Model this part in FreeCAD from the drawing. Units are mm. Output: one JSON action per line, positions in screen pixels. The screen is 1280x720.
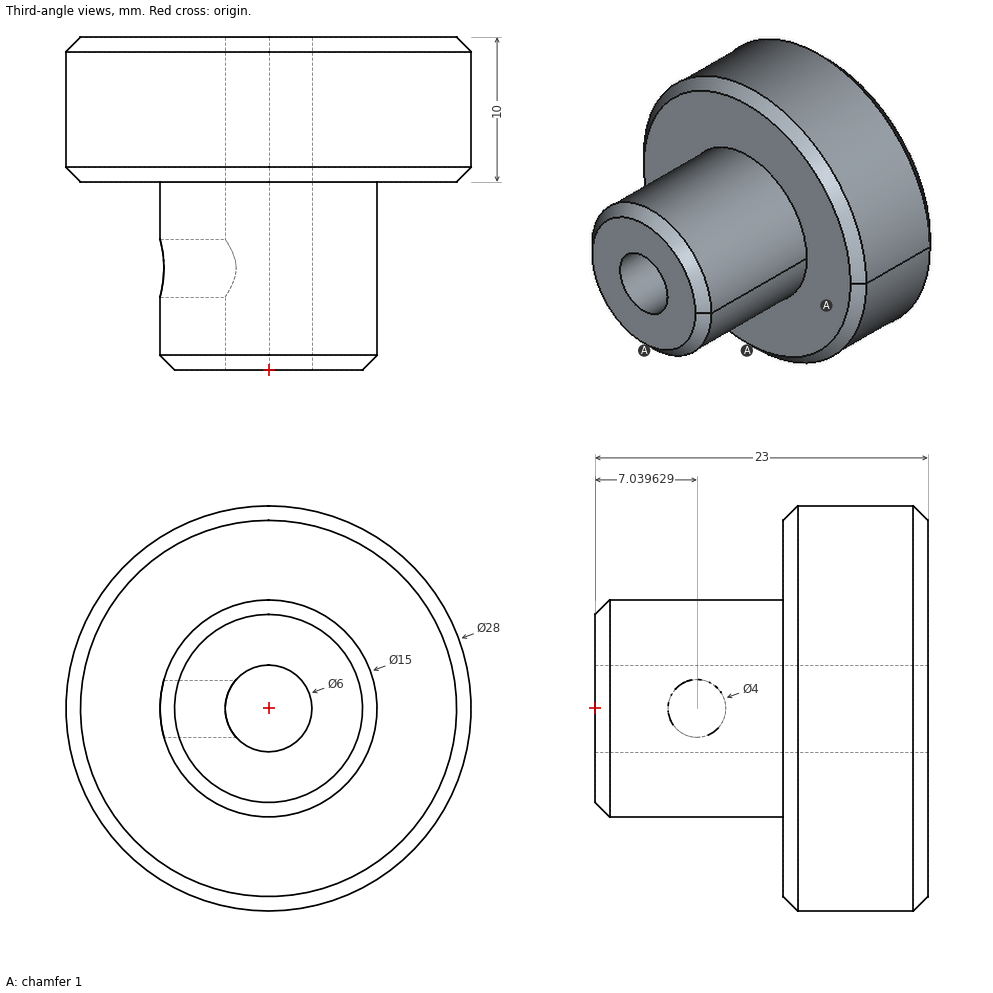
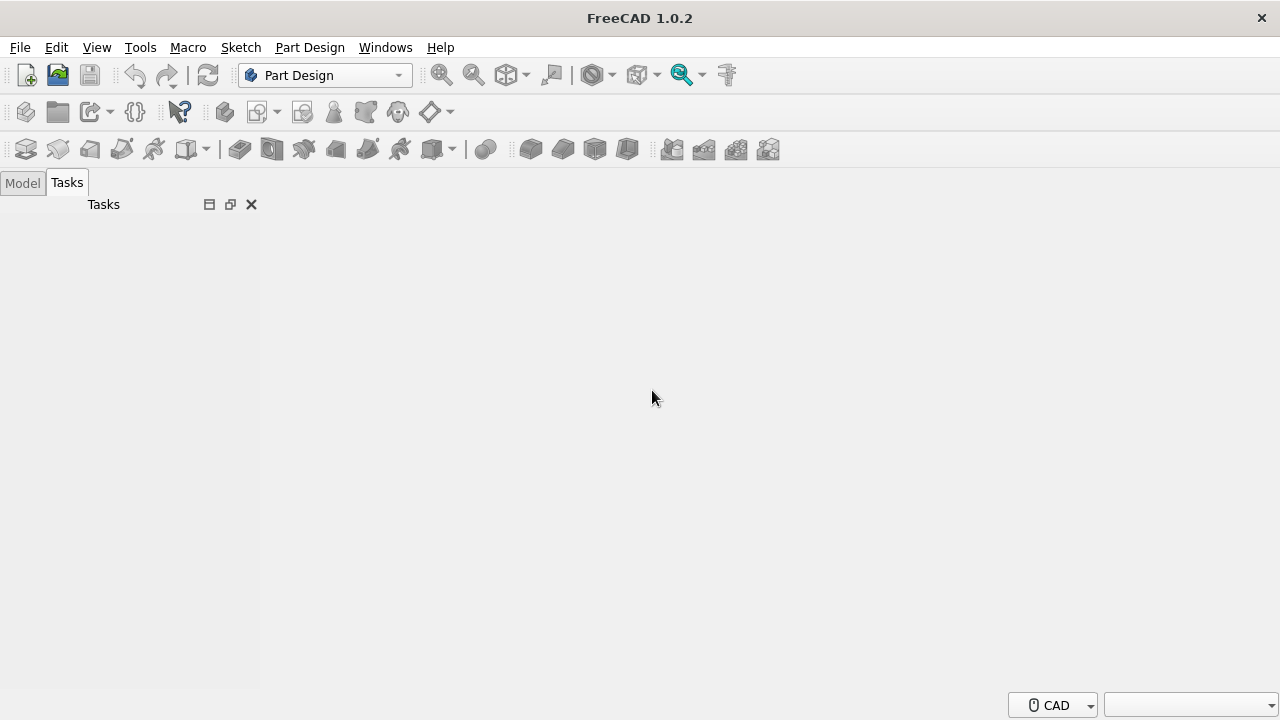
{"action": "left_click", "coordinate": [26, 76]}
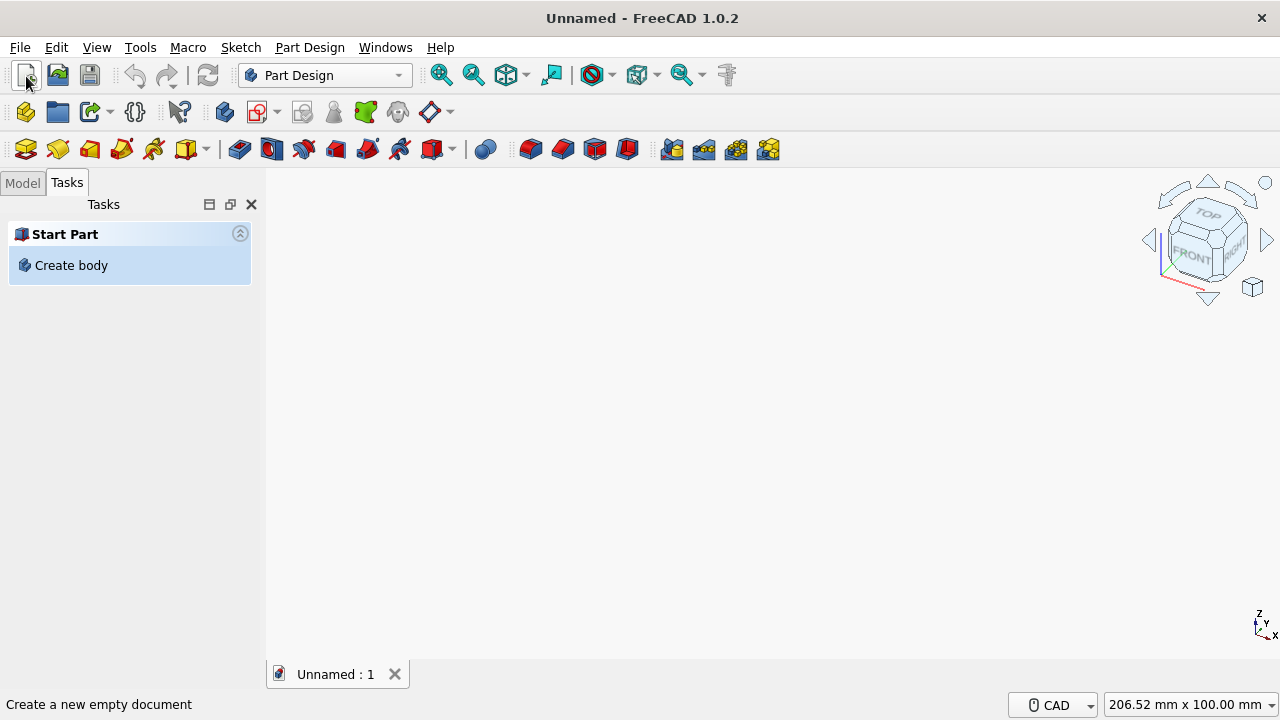
{"action": "left_click", "coordinate": [258, 112]}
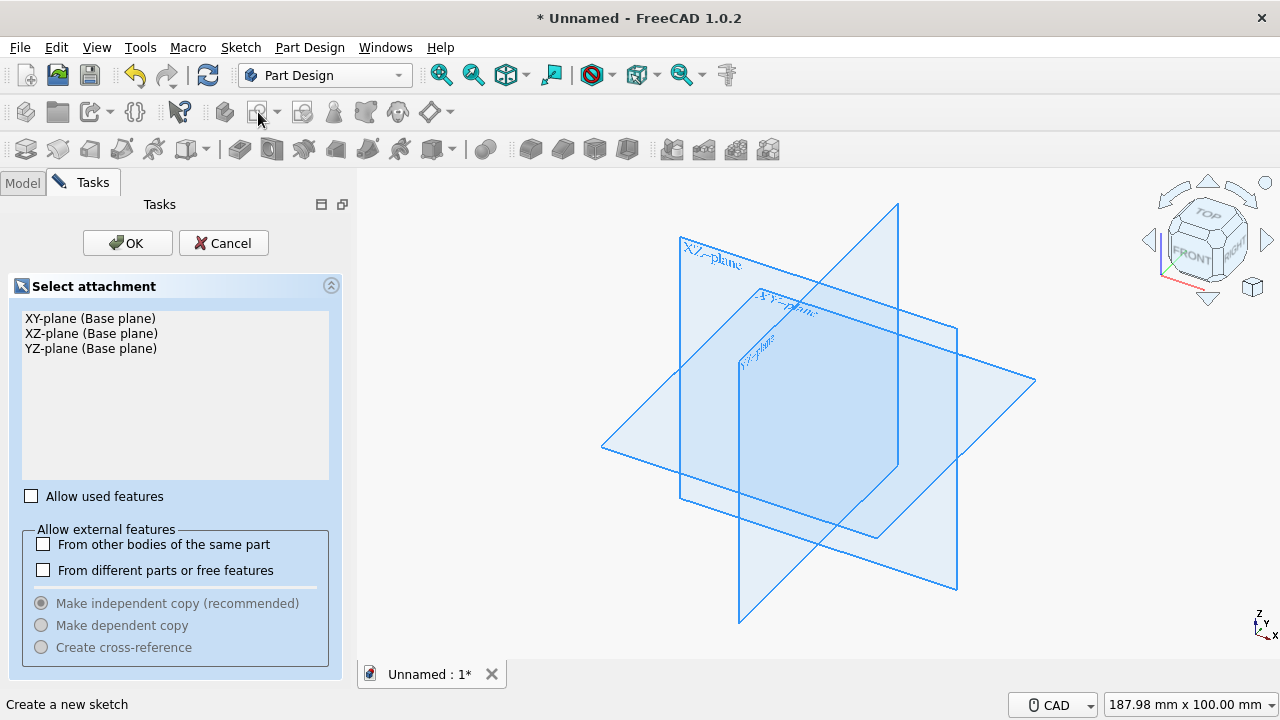
{"action": "left_click", "coordinate": [82, 334]}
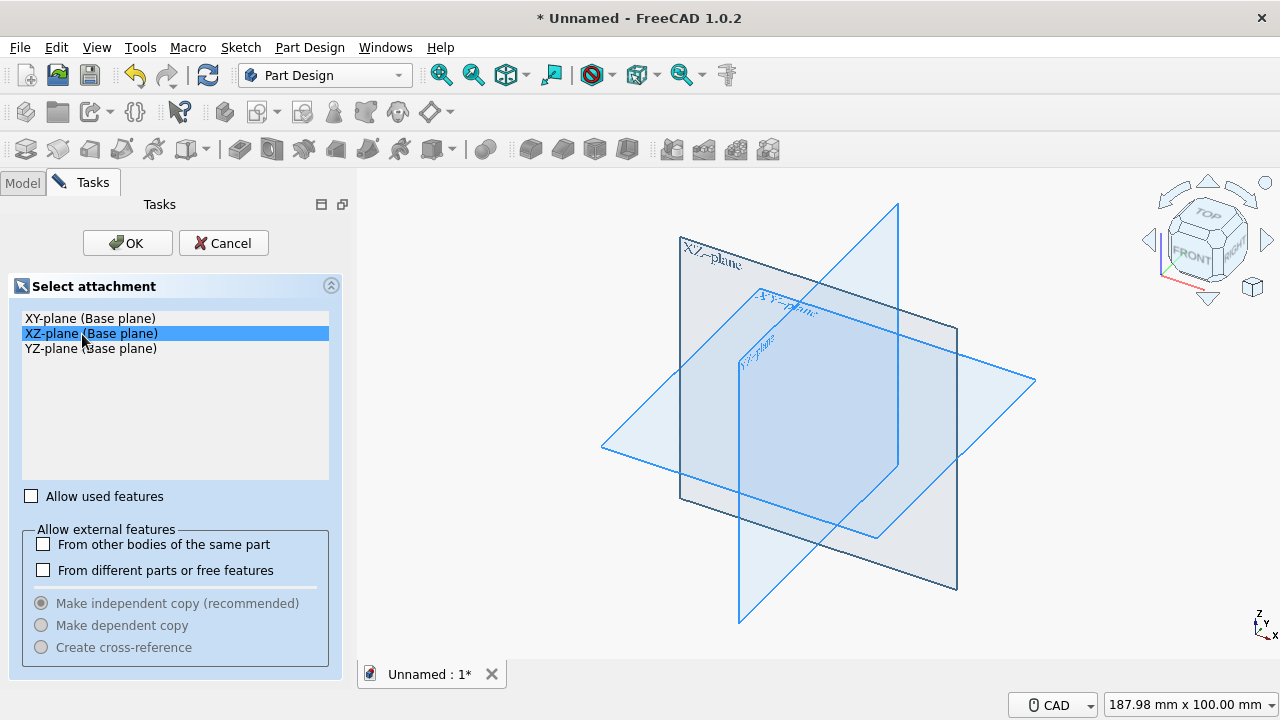
{"action": "left_click", "coordinate": [128, 243]}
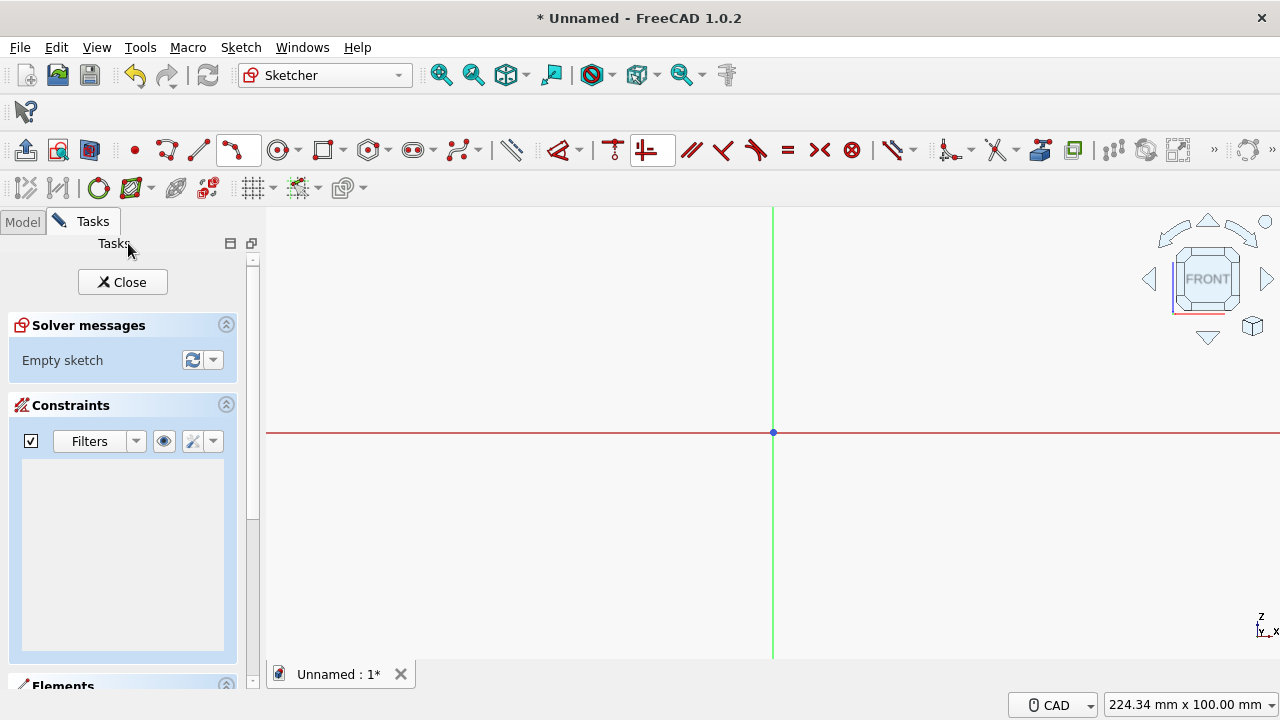
{"action": "scroll", "coordinate": [795, 433], "scroll_direction": "up", "scroll_amount": 7}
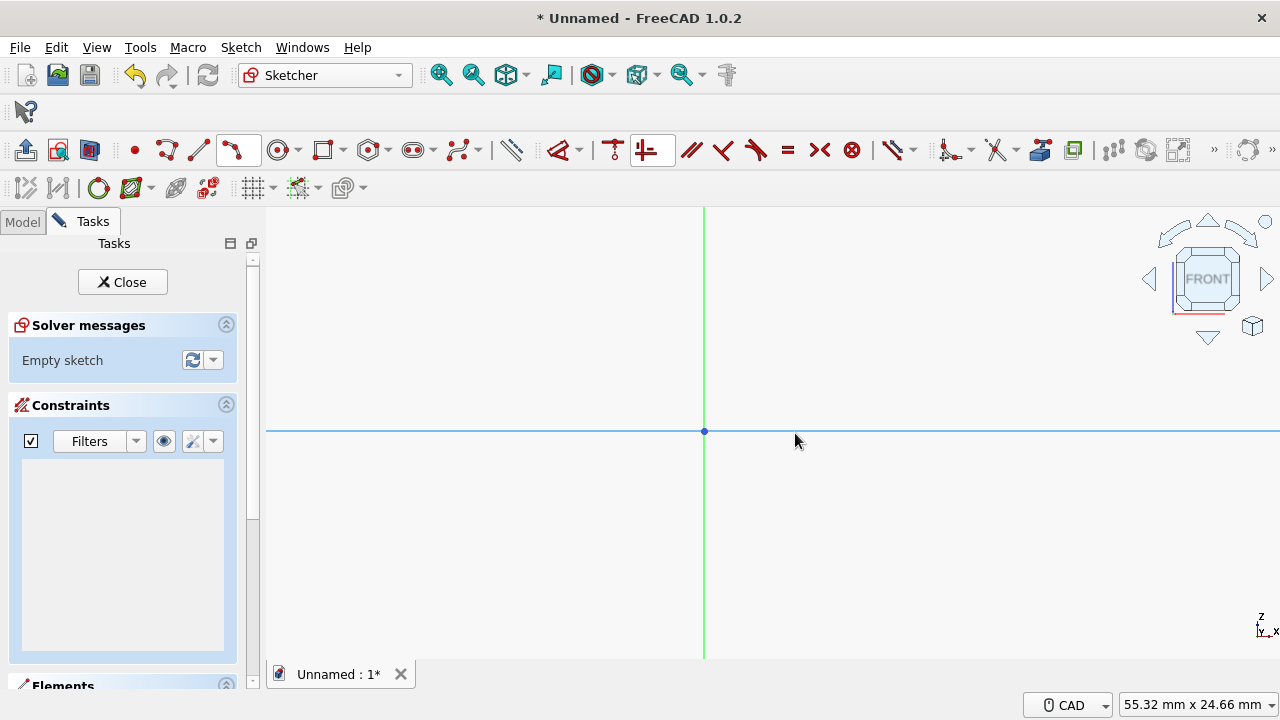
{"action": "left_click", "coordinate": [278, 150]}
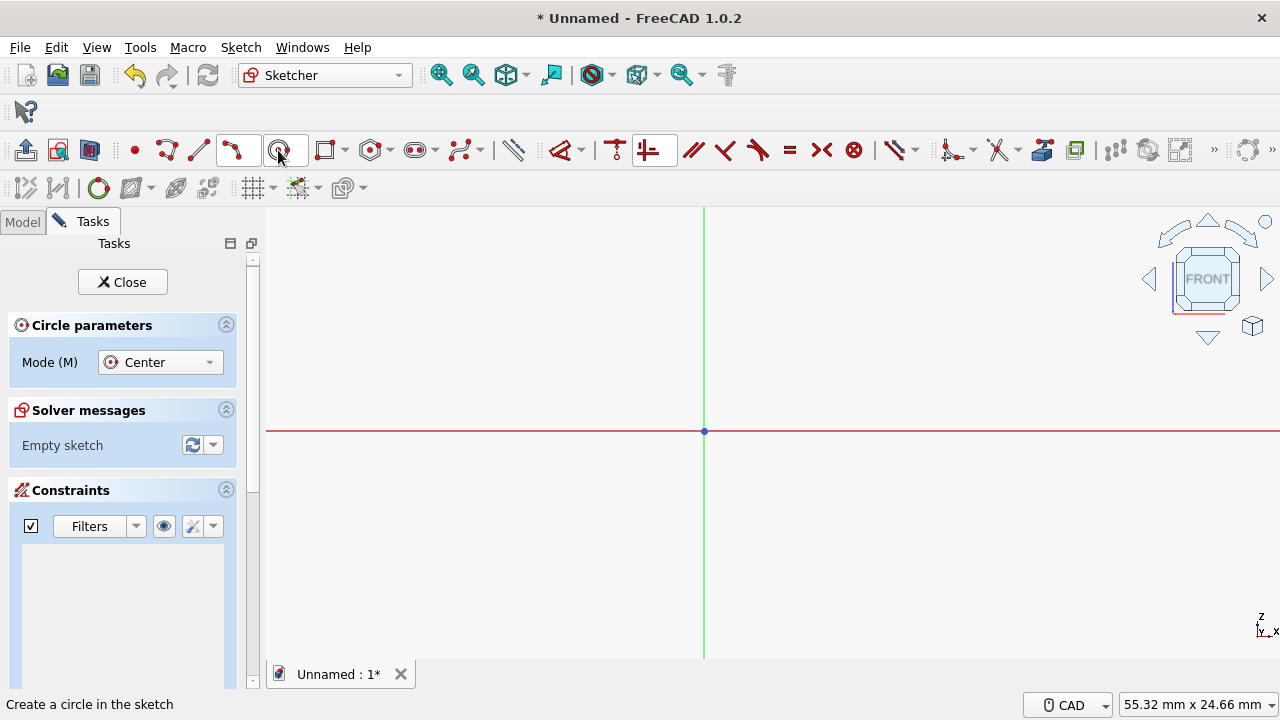
{"action": "left_click", "coordinate": [704, 431]}
{"action": "mouse_move", "coordinate": [801, 334]}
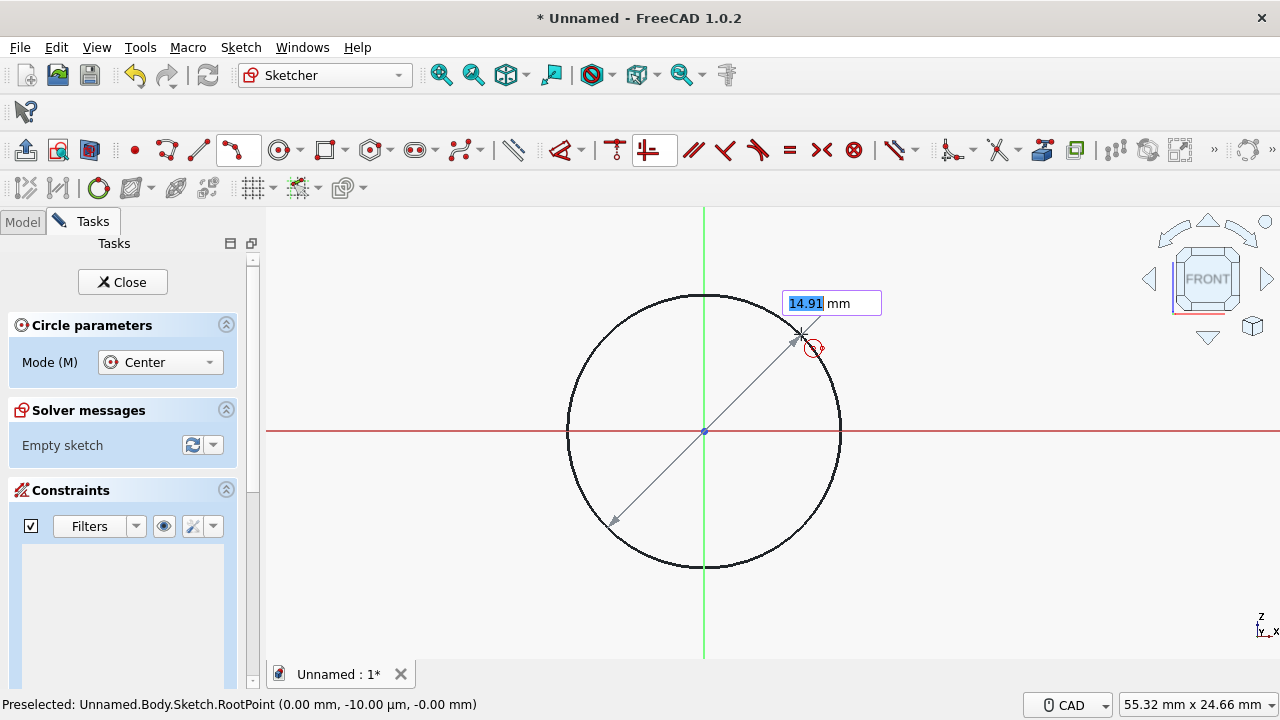
{"action": "type", "text": "15"}
{"action": "key", "text": "Return"}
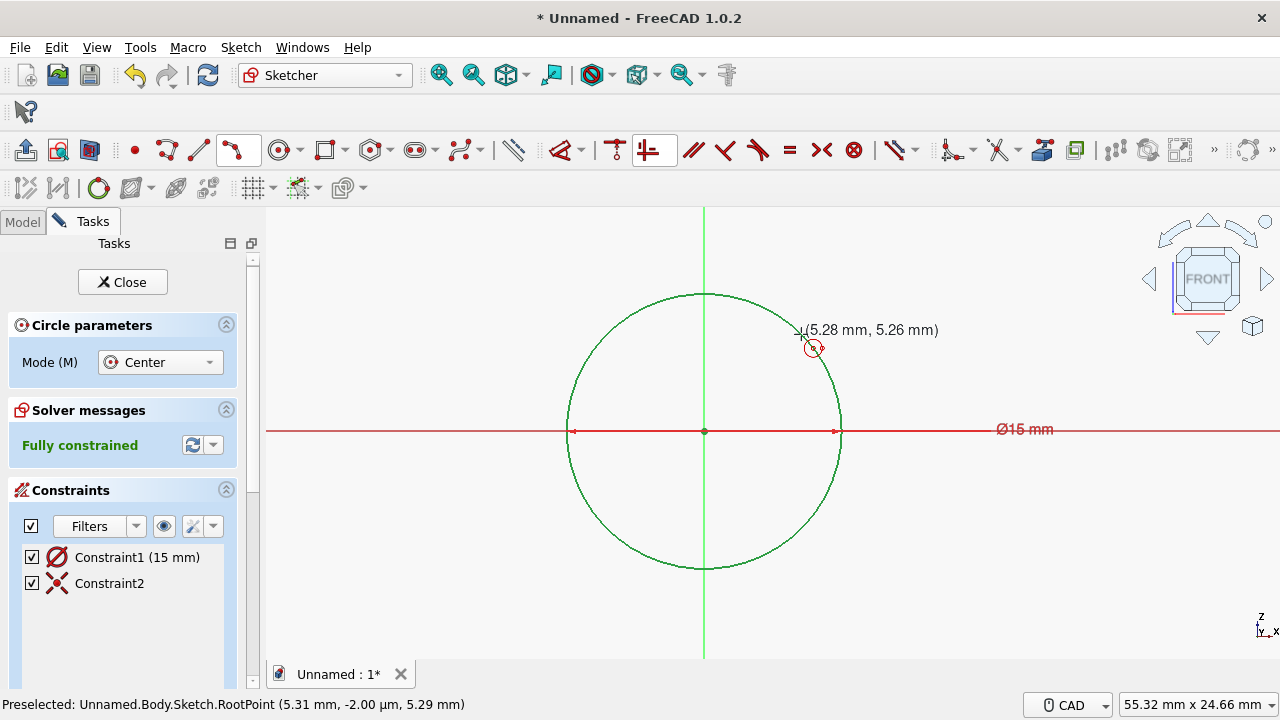
{"action": "left_click", "coordinate": [704, 431]}
{"action": "mouse_move", "coordinate": [743, 393]}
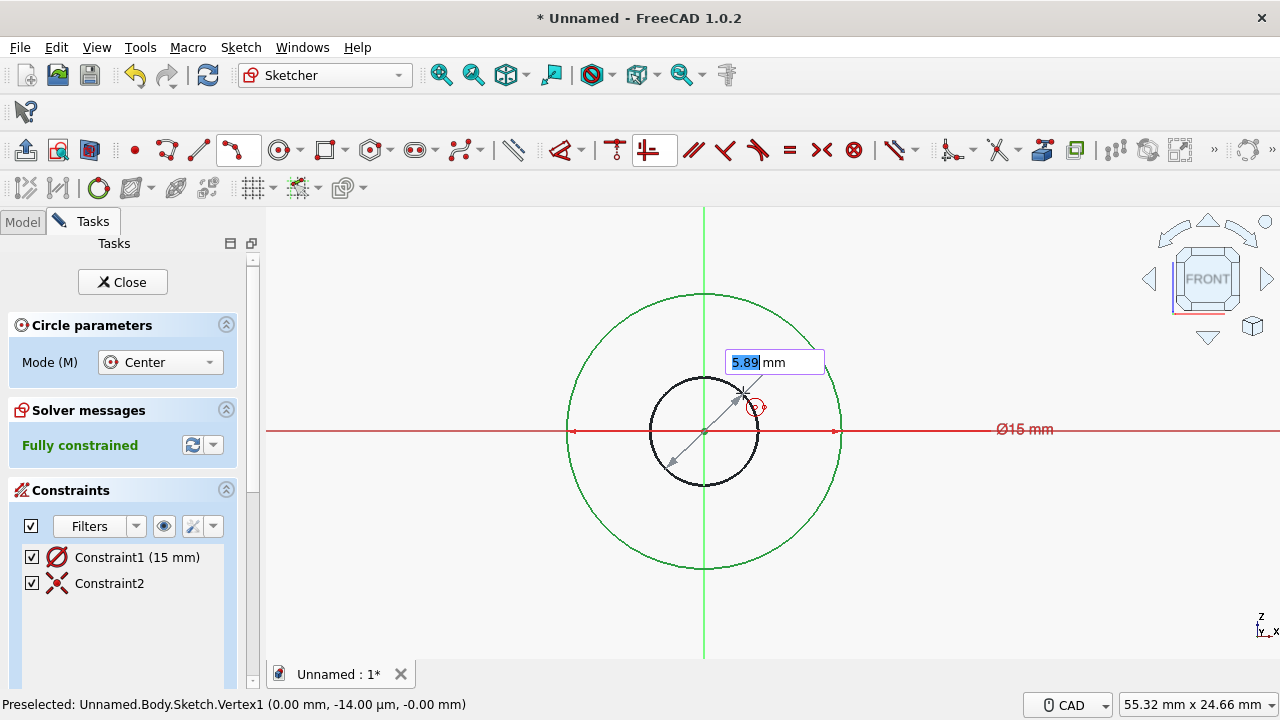
{"action": "type", "text": "6"}
{"action": "key", "text": "Return"}
{"action": "key", "text": "Escape"}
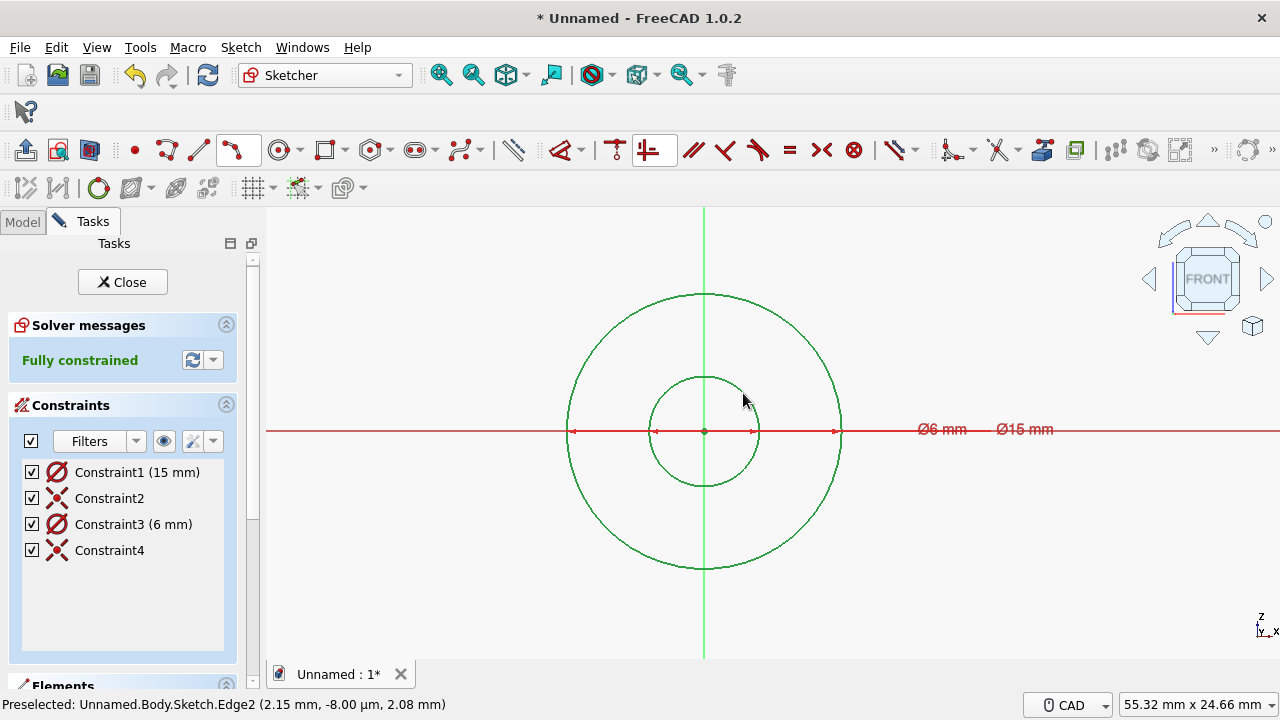
{"action": "left_click", "coordinate": [123, 282]}